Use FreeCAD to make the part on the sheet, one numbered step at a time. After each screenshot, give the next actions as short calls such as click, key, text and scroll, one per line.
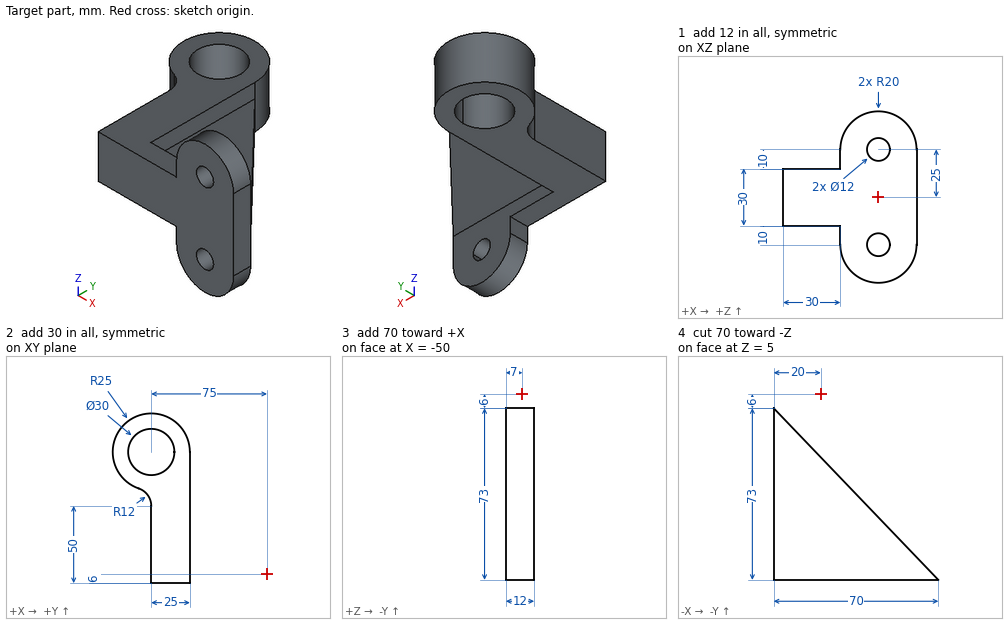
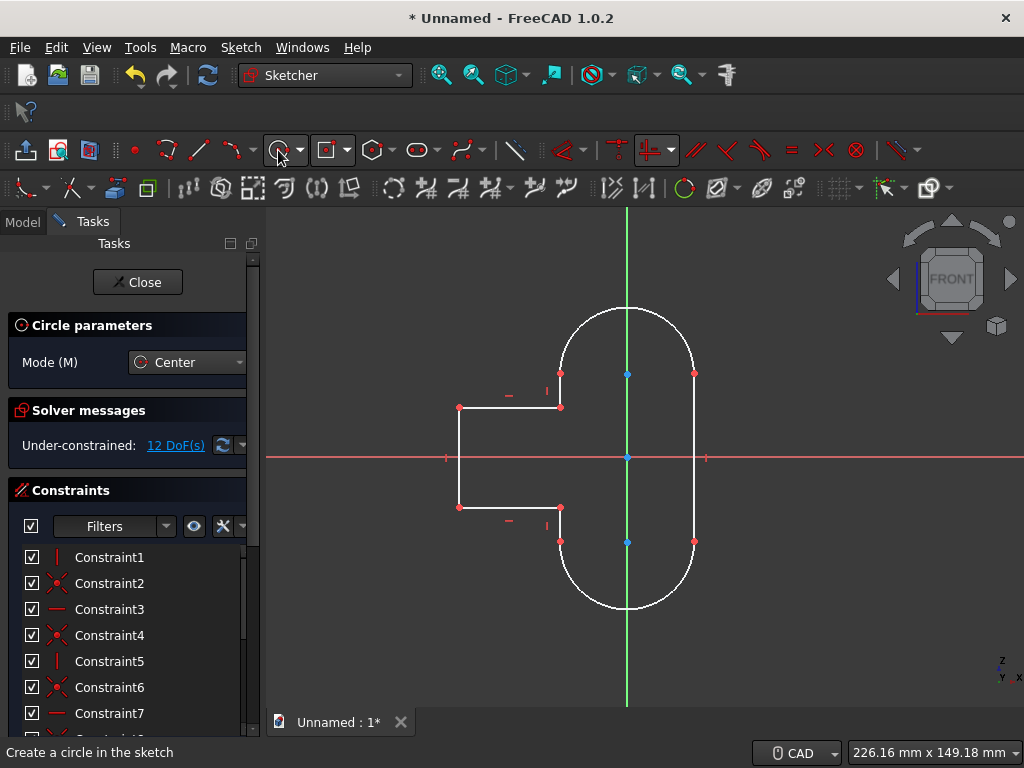
click(627, 373)
click(641, 359)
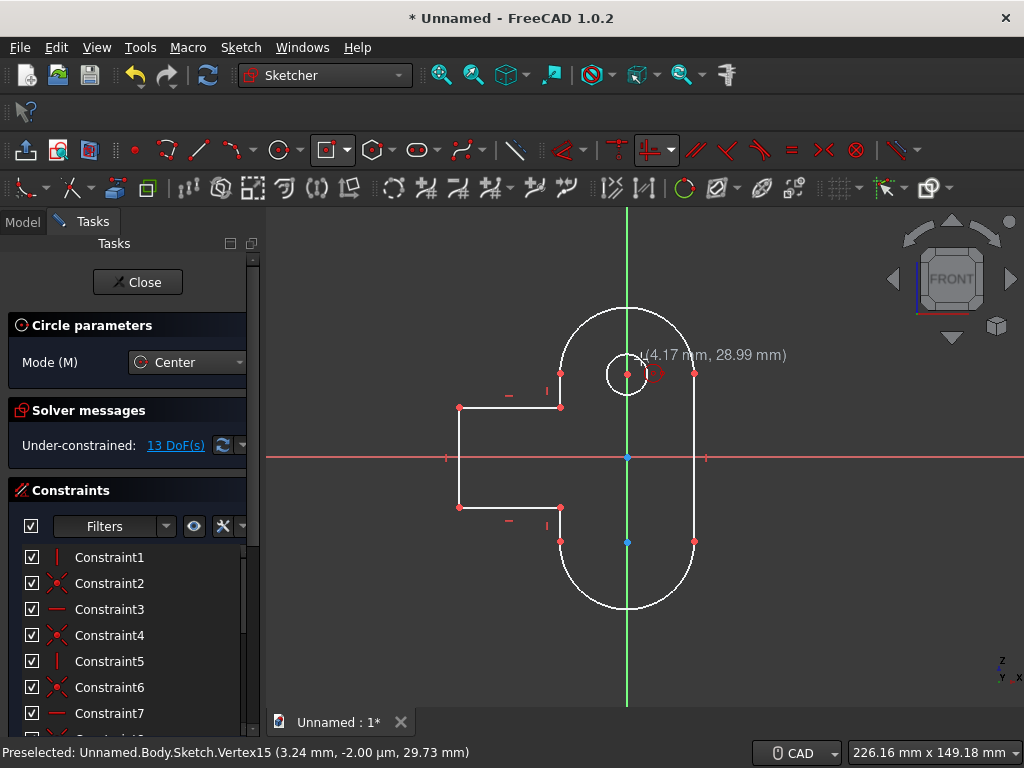
click(627, 541)
click(641, 527)
key(Escape)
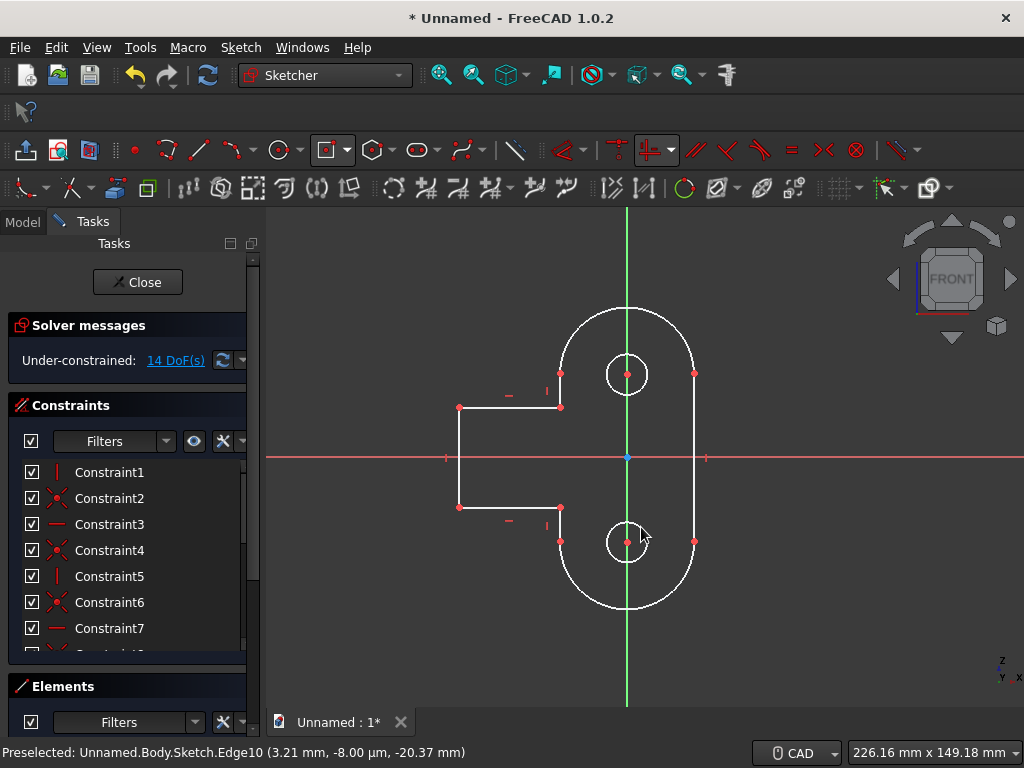
scroll(560, 532, up, 2)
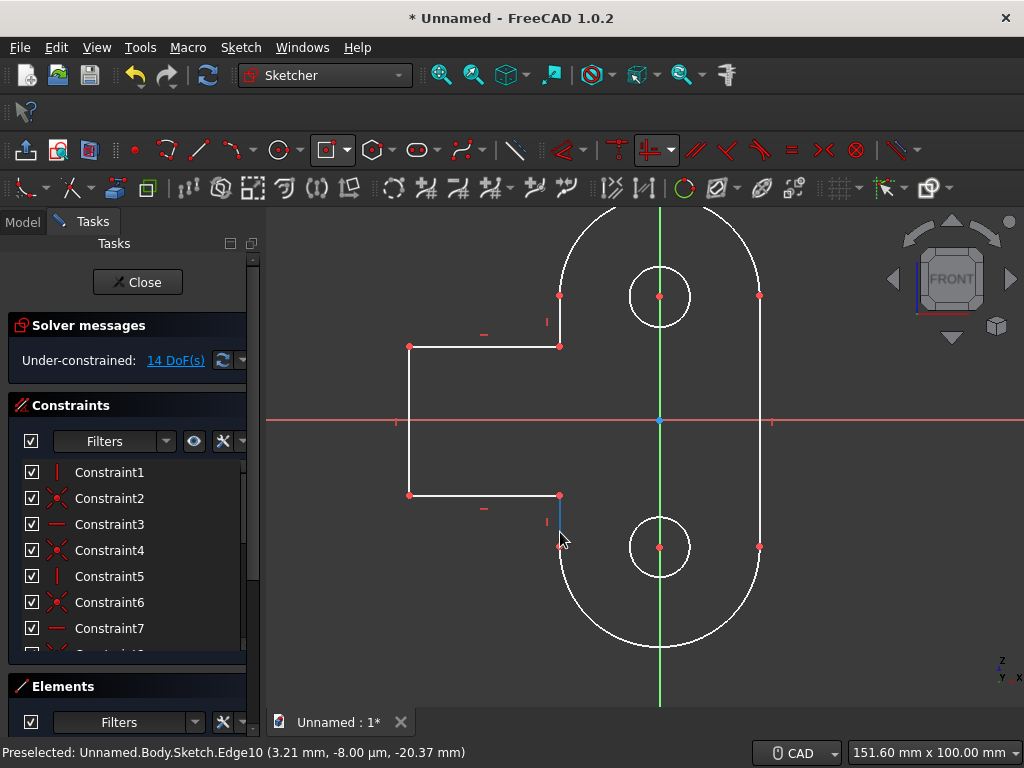
click(560, 531)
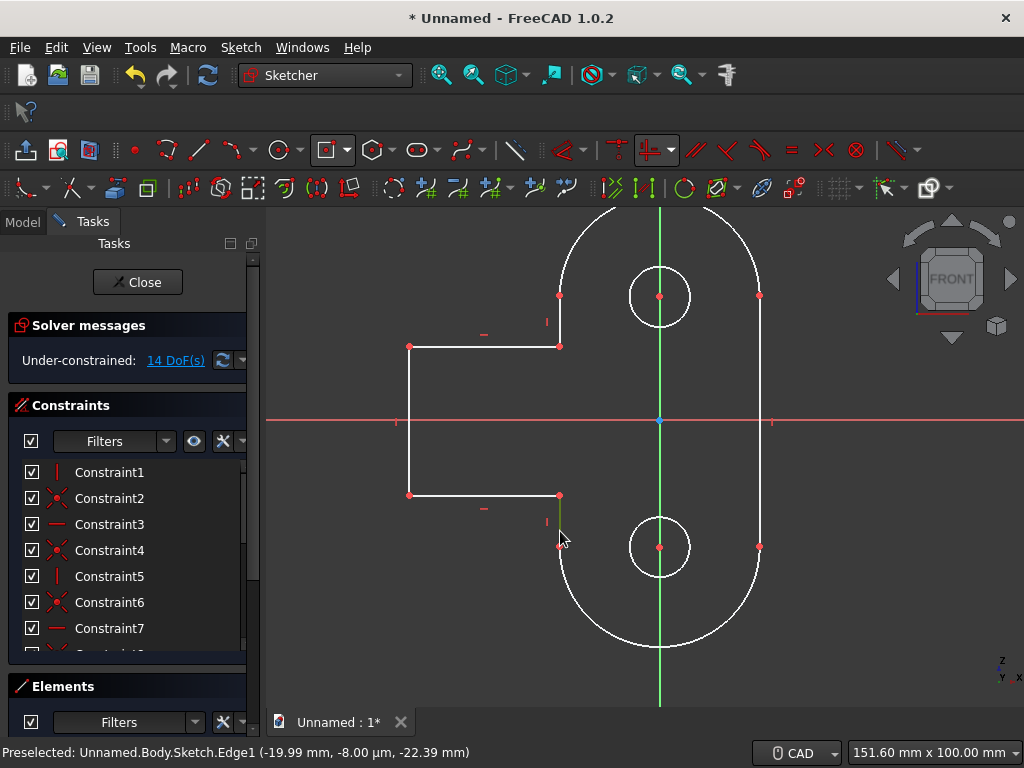
click(601, 628)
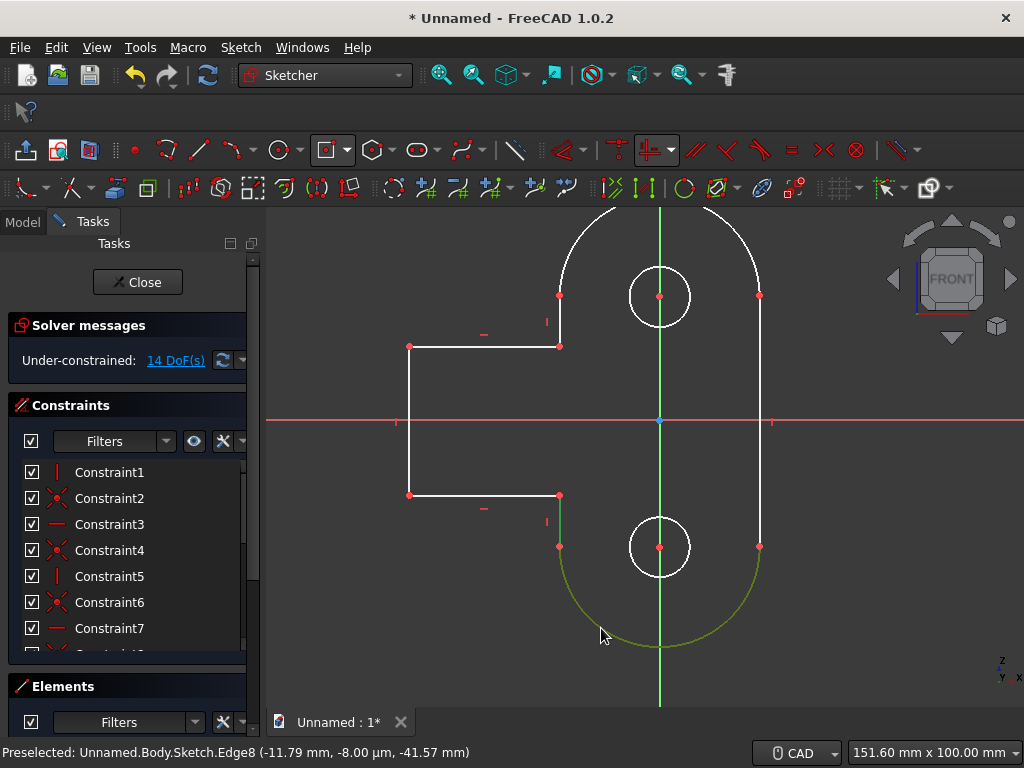
click(760, 150)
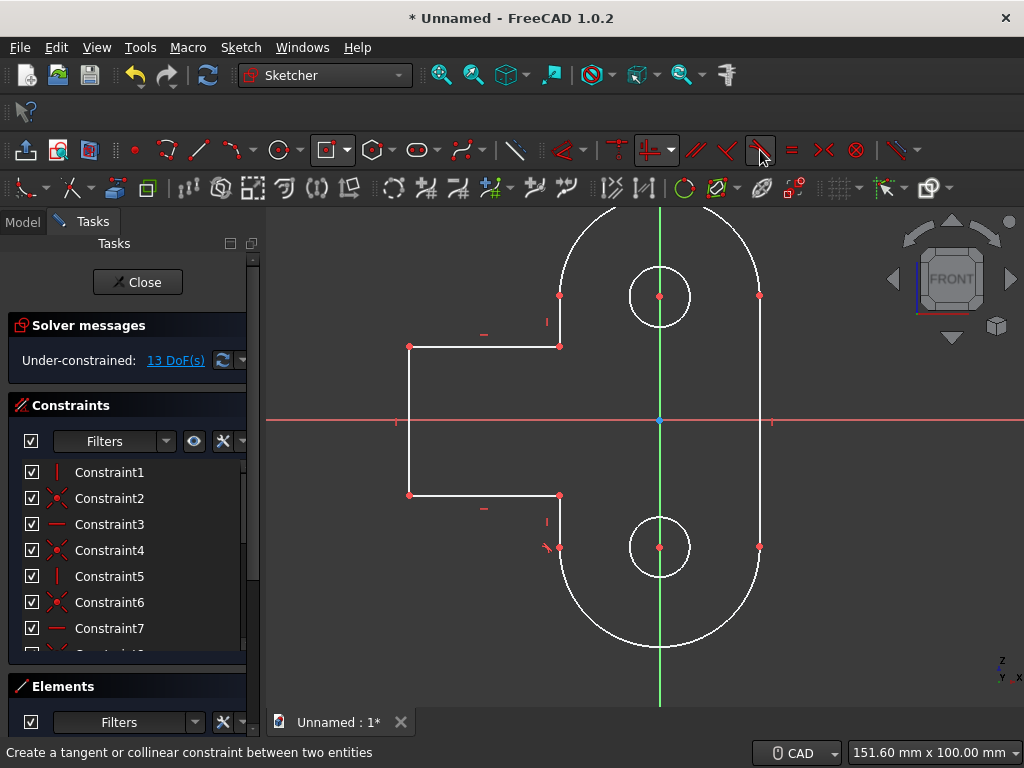
click(560, 331)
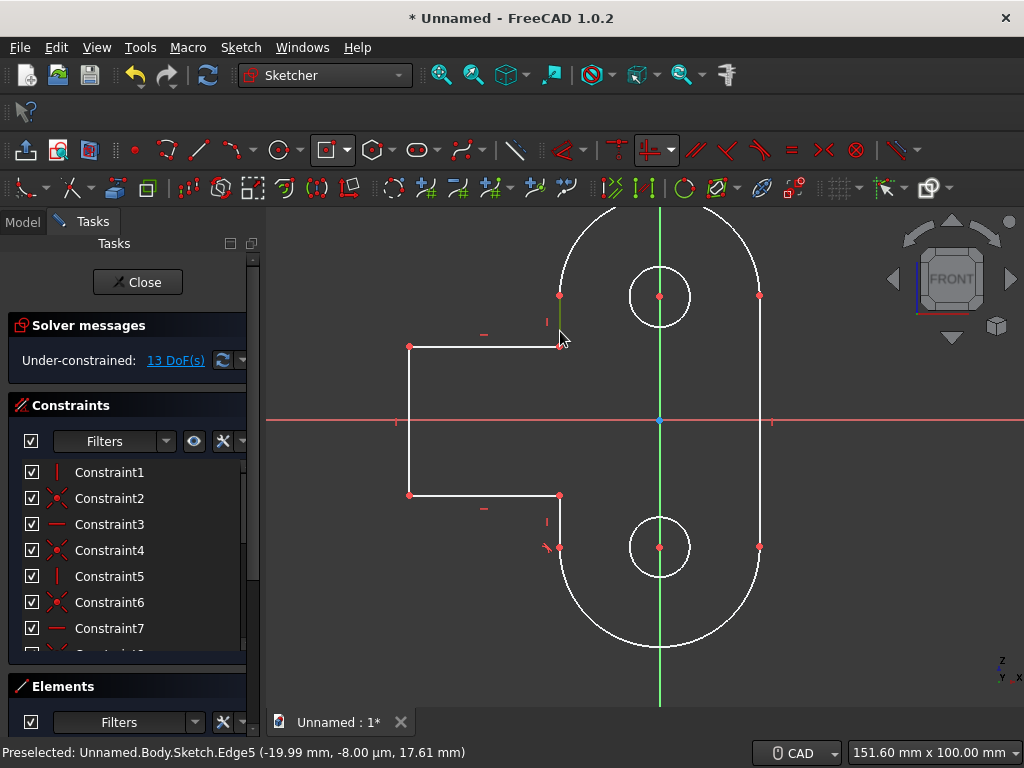
click(740, 238)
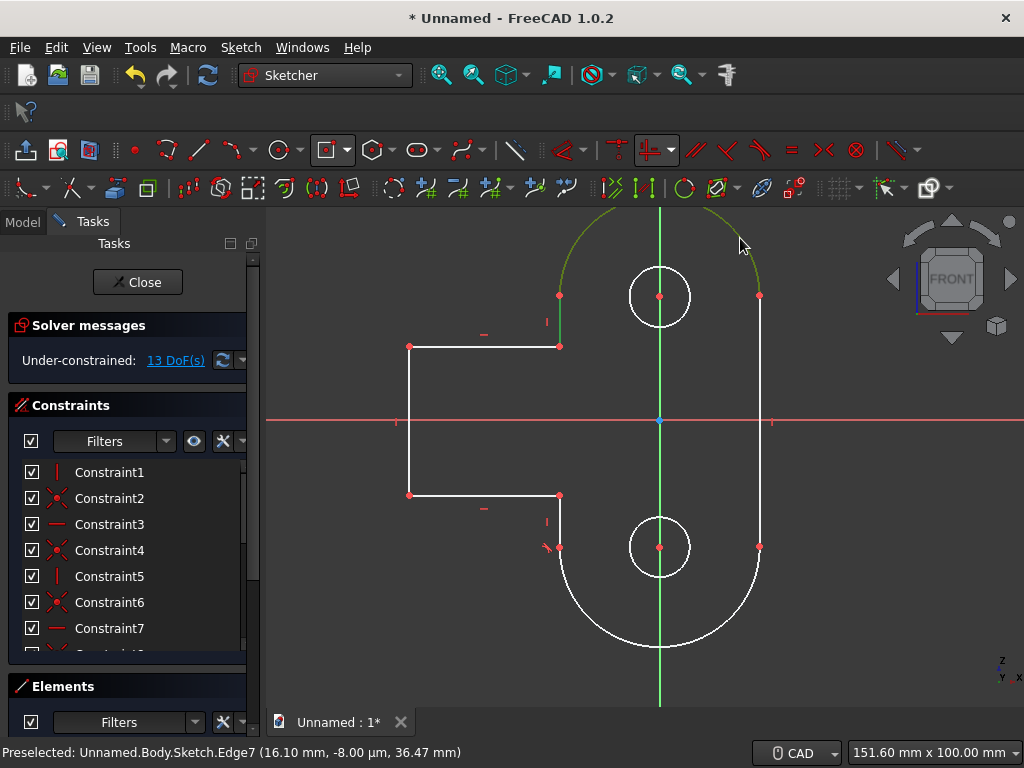
click(760, 150)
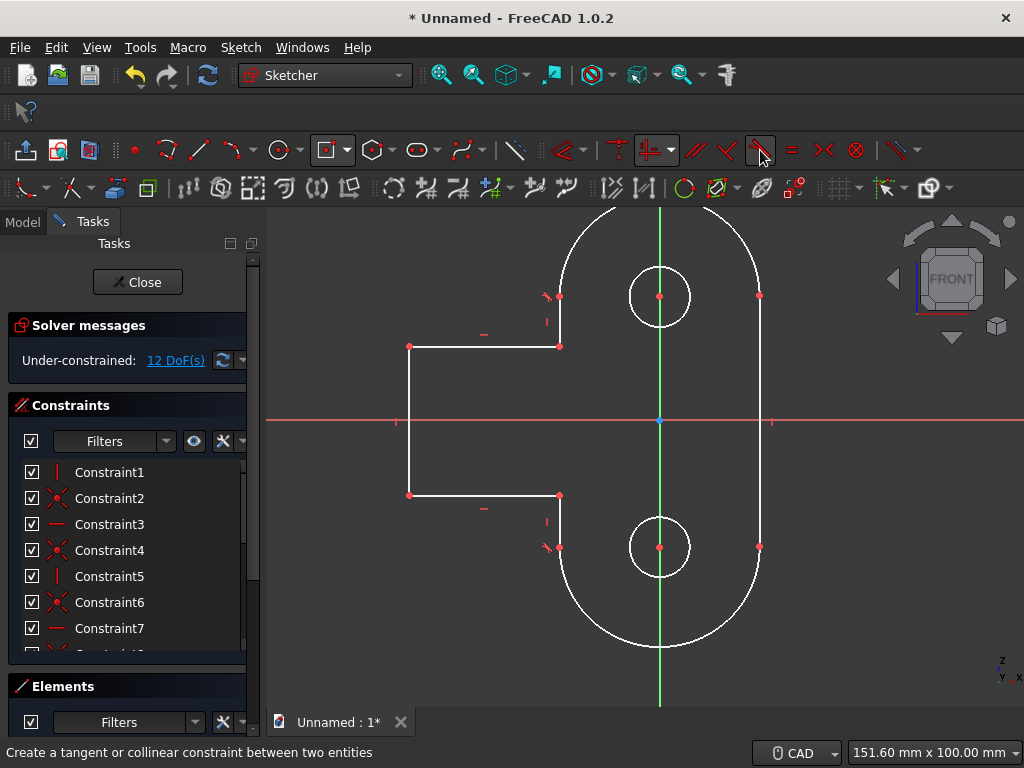
click(760, 371)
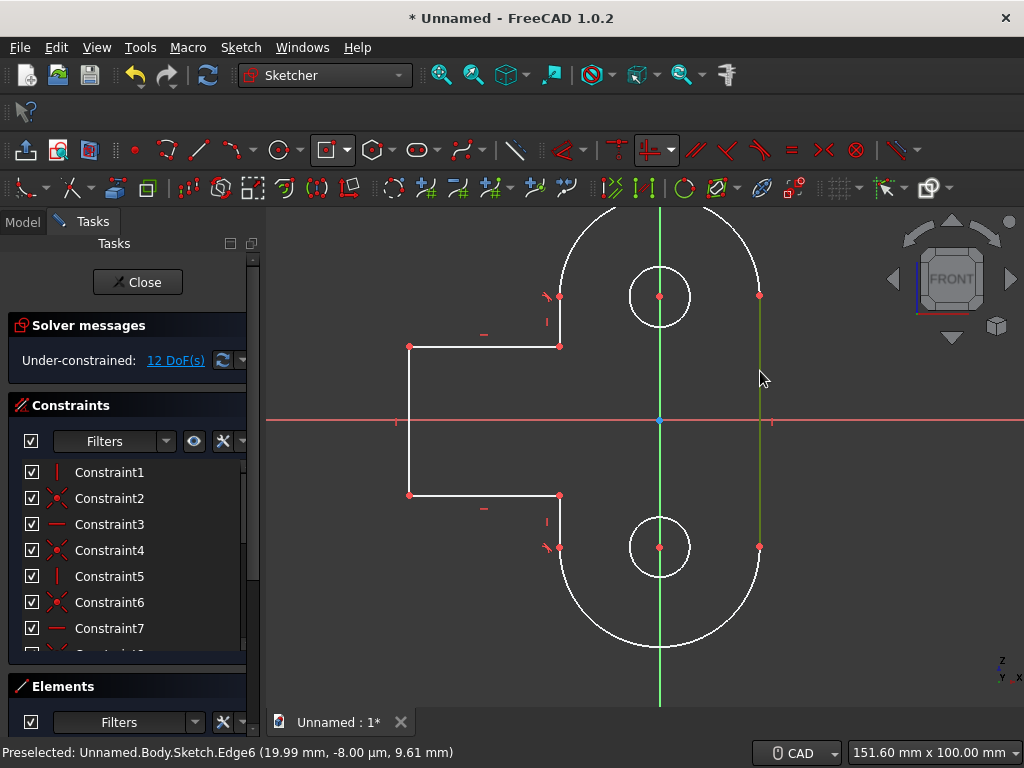
click(740, 238)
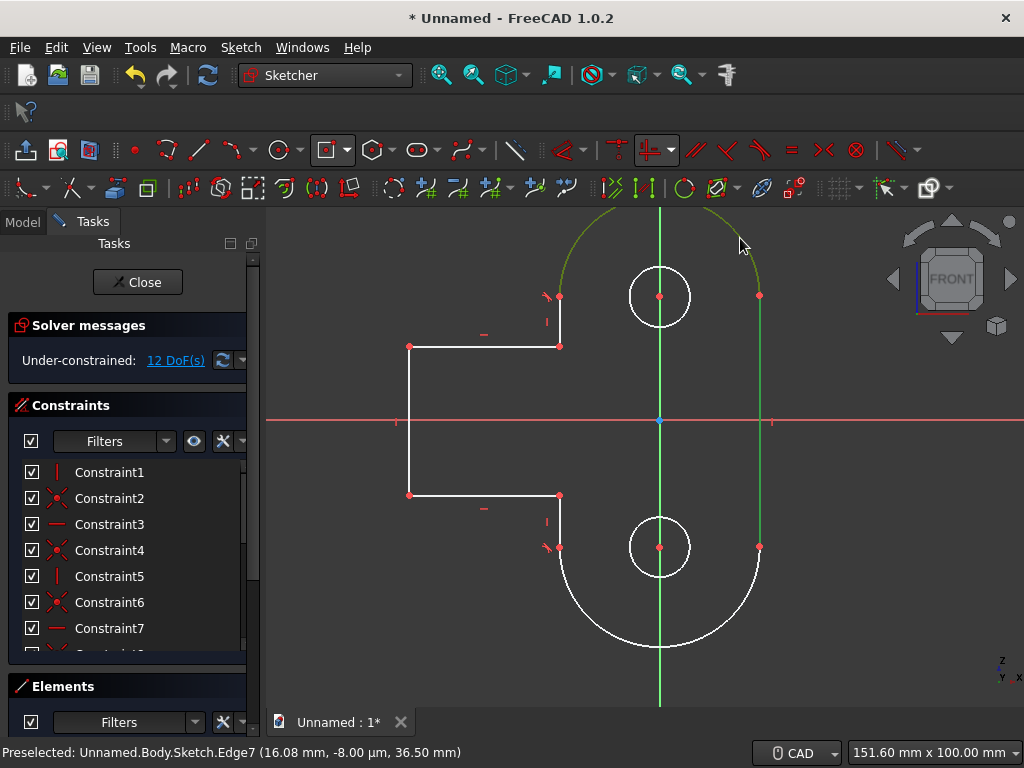
click(760, 150)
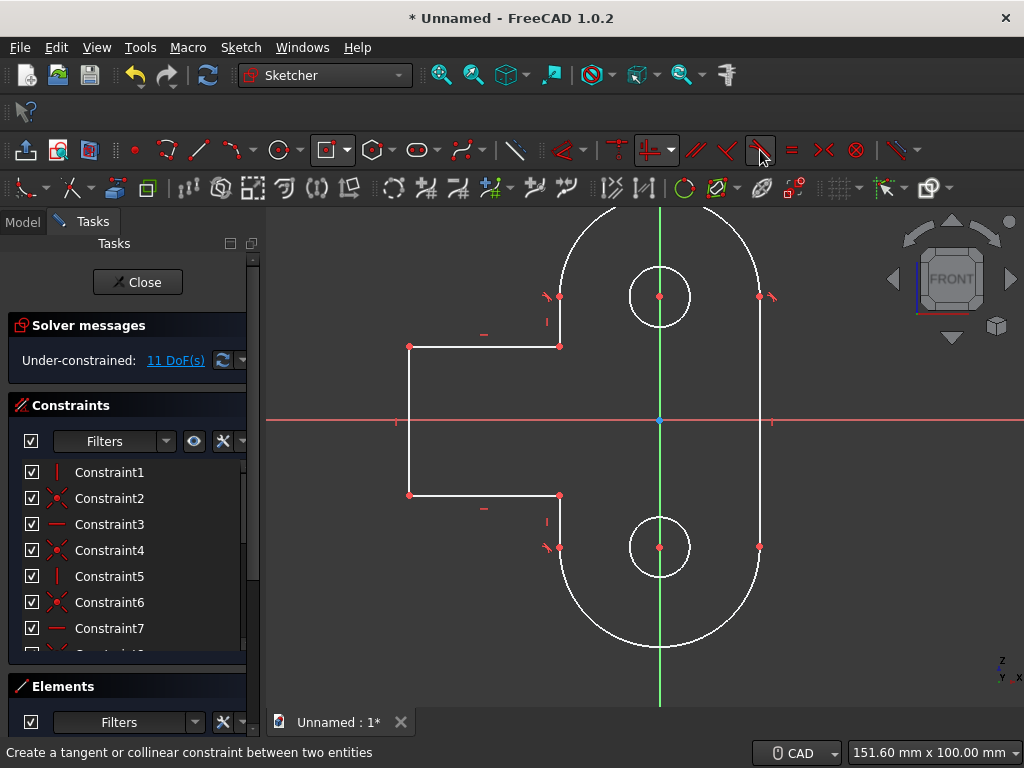
click(760, 372)